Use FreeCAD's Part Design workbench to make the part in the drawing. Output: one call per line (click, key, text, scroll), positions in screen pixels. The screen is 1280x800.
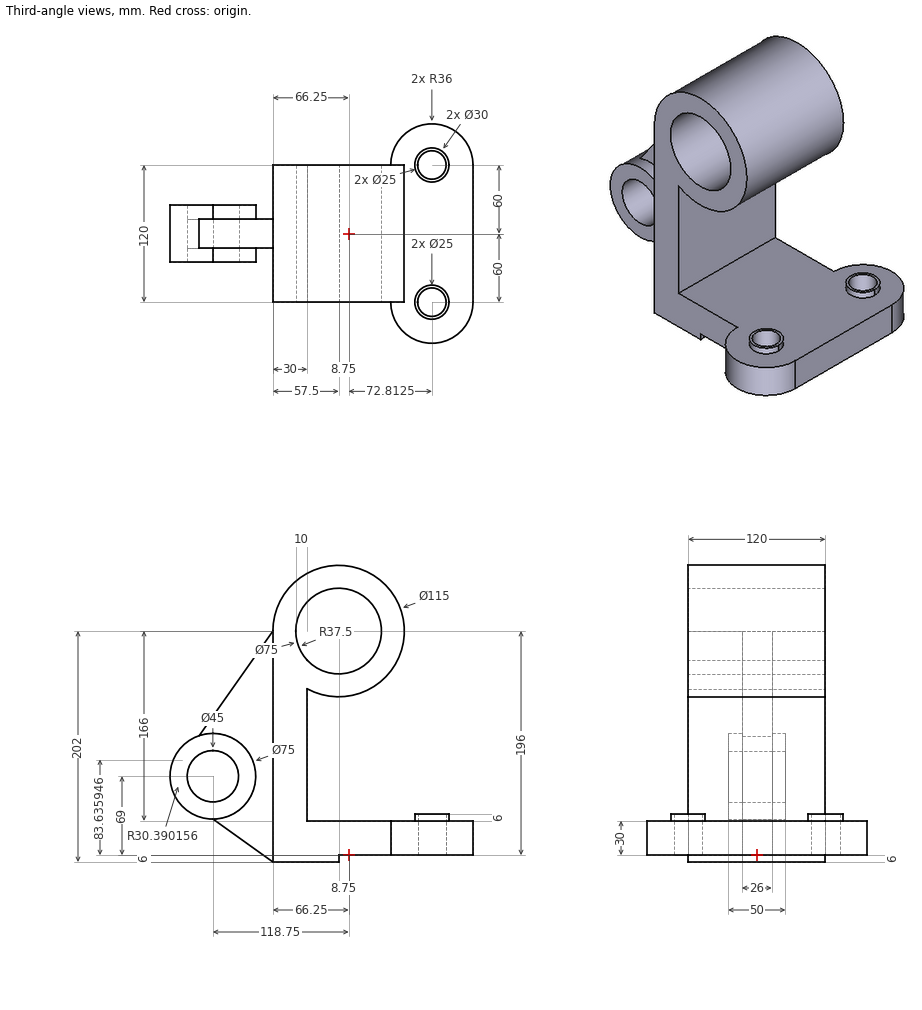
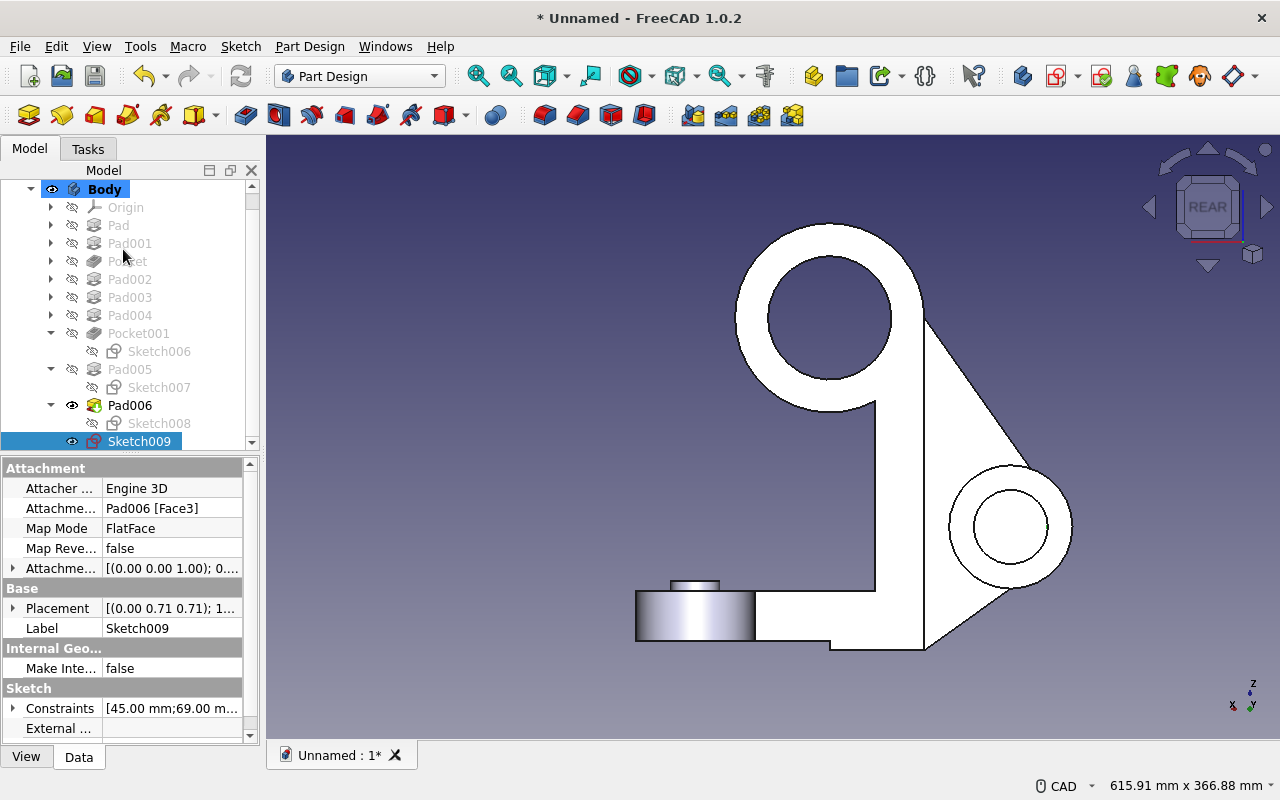
click(246, 116)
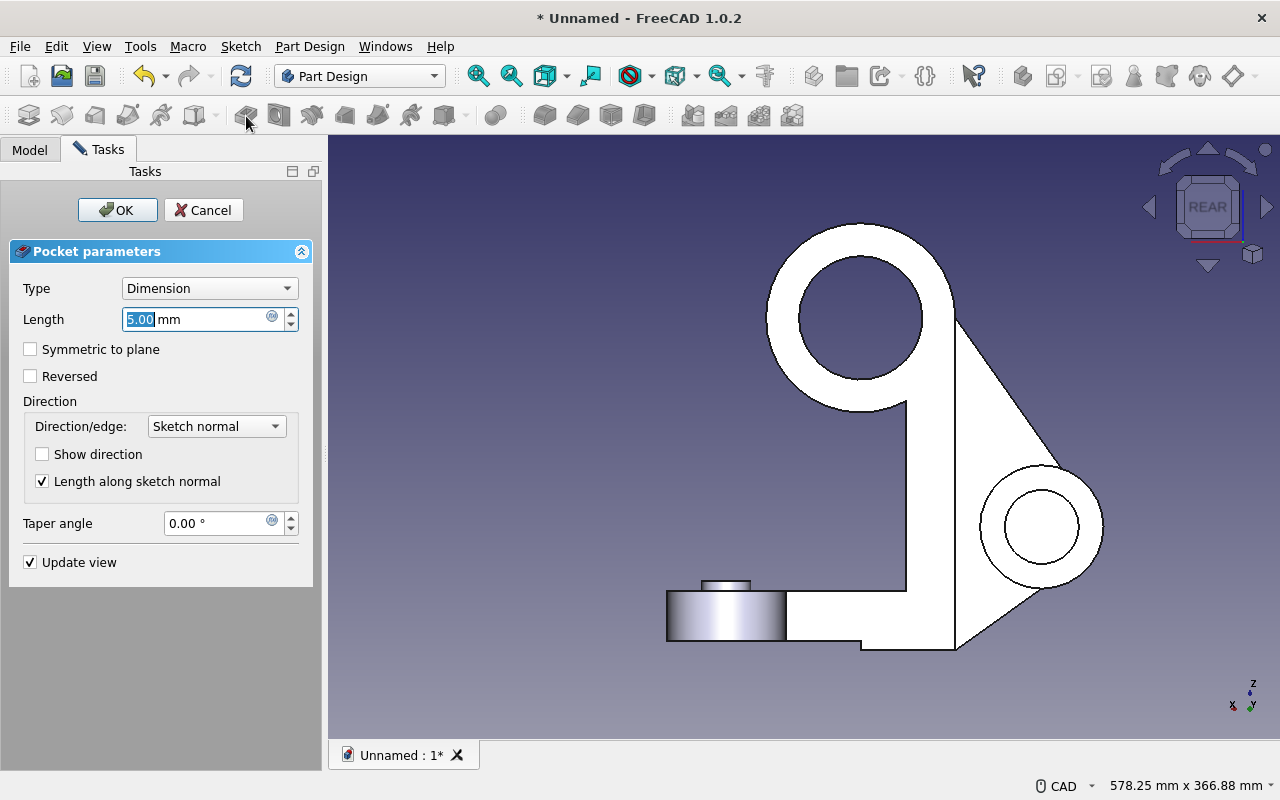
click(210, 288)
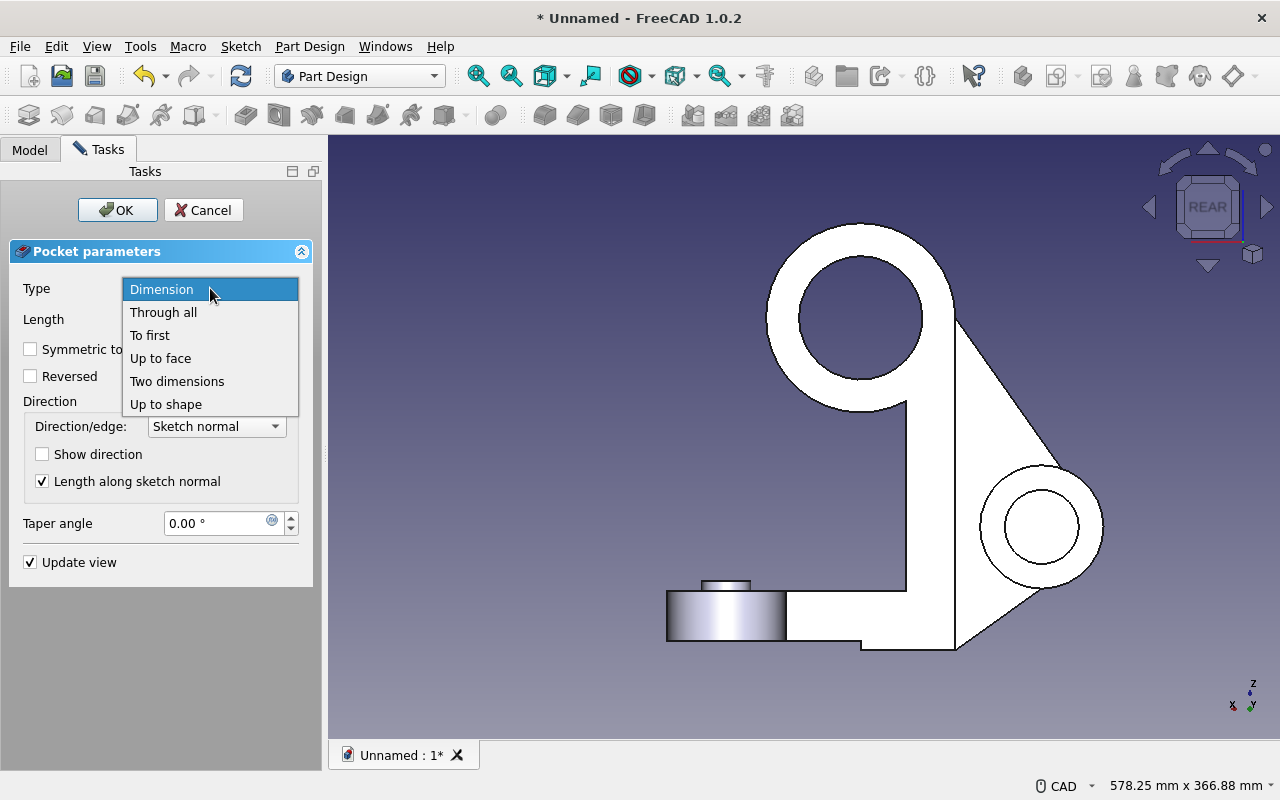
click(208, 312)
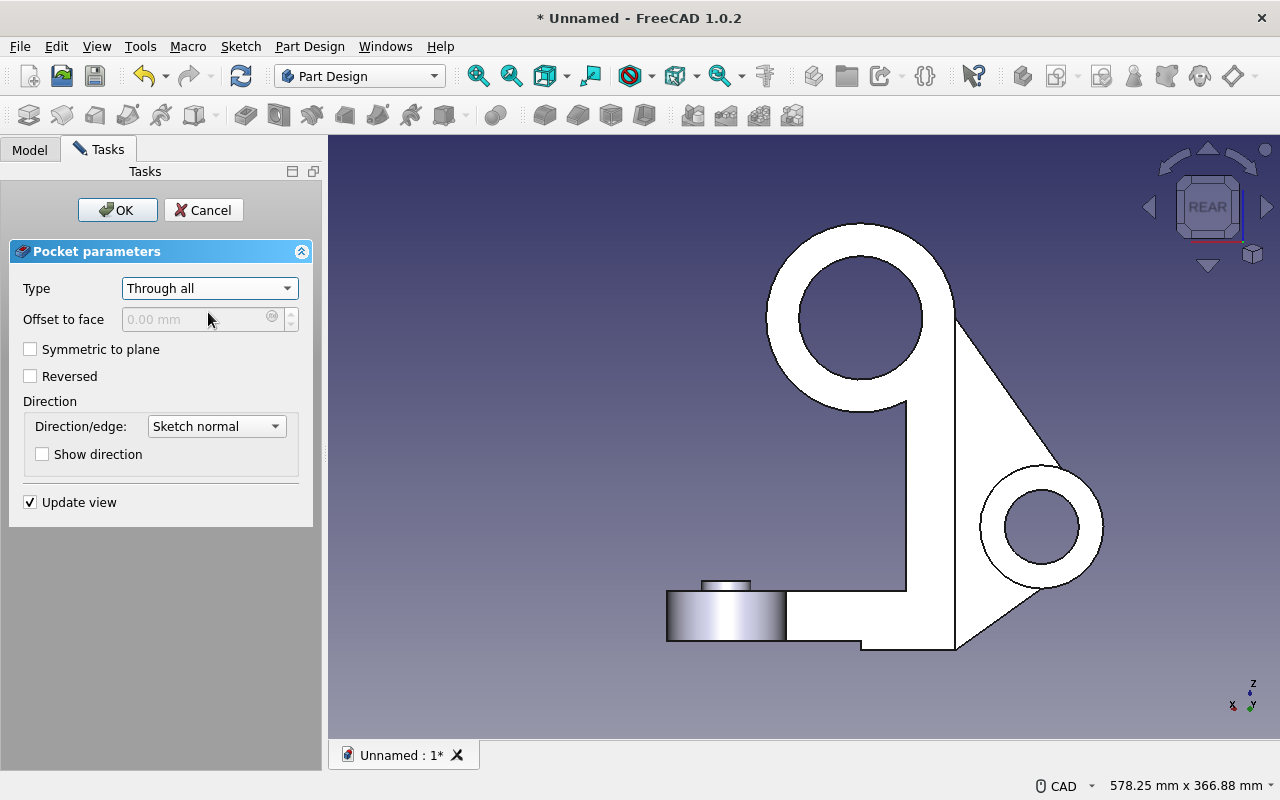
click(118, 210)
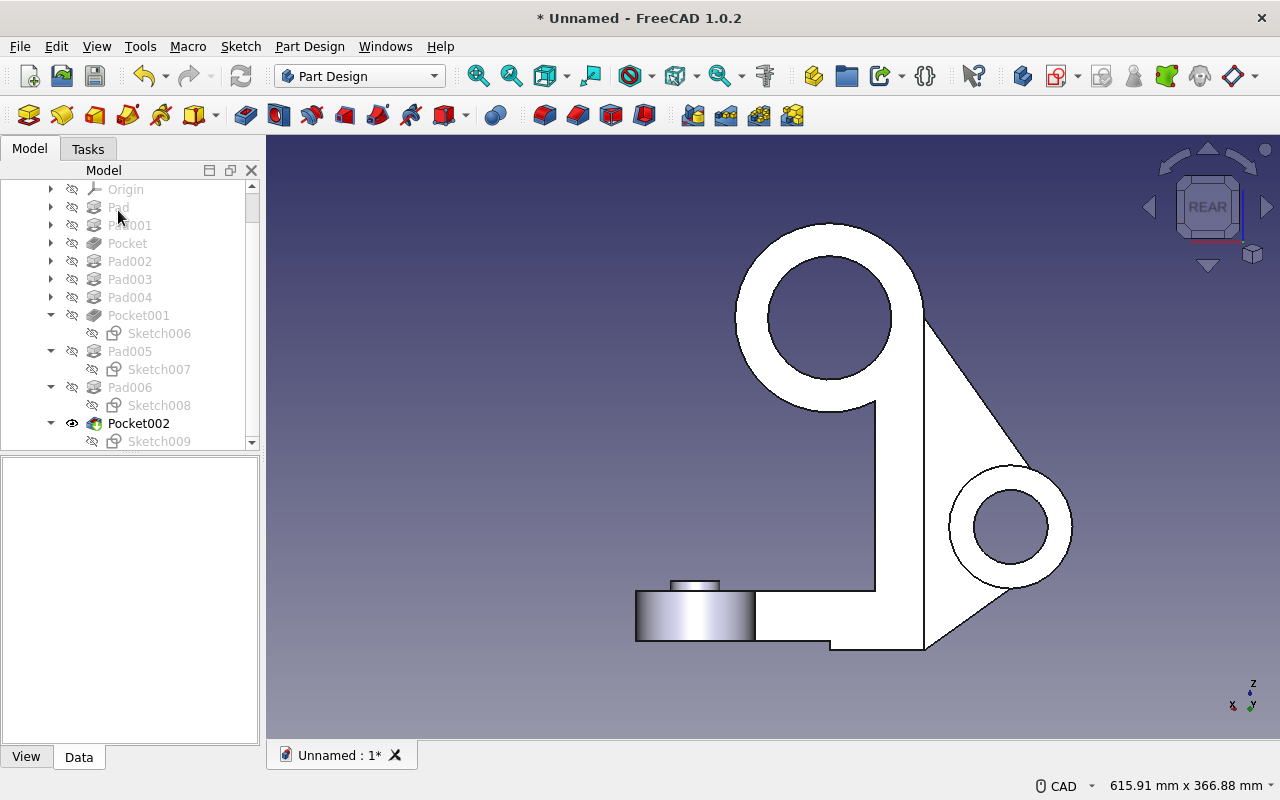
key(0)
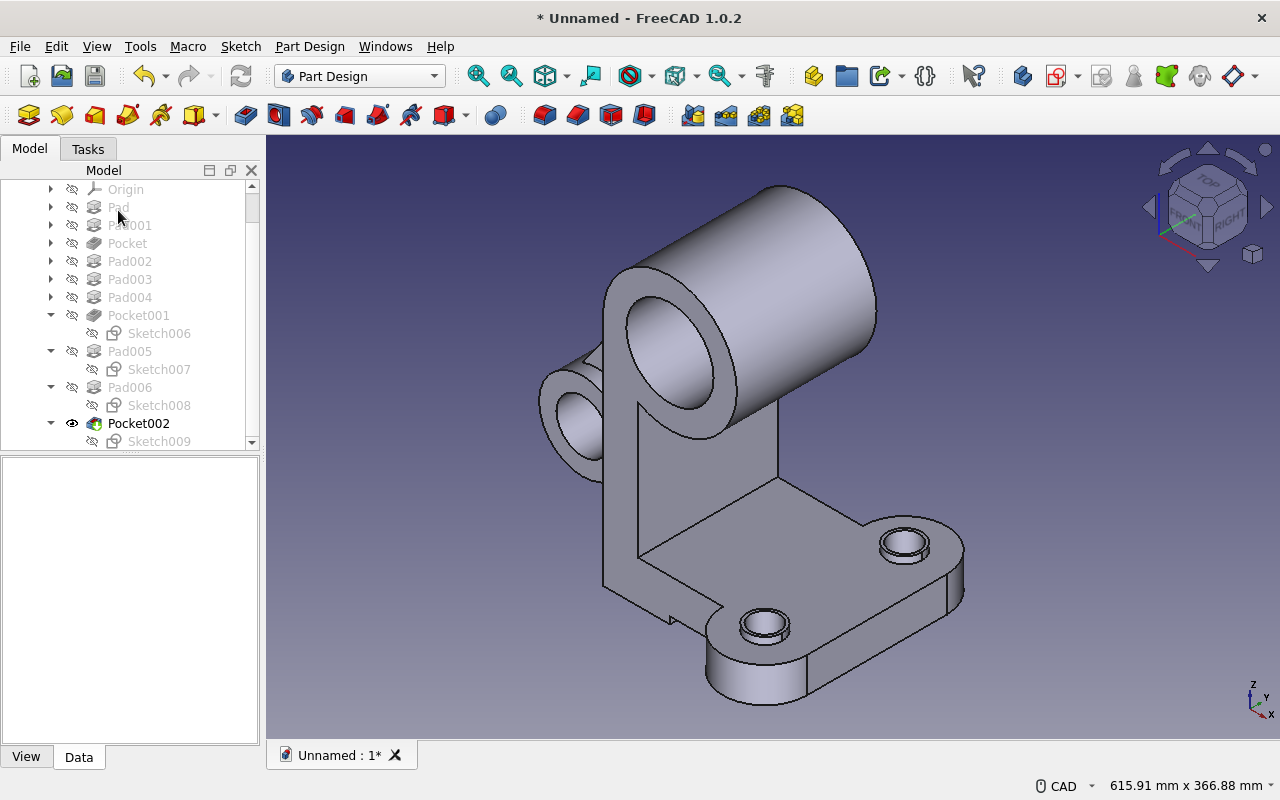
key(v)
key(f)